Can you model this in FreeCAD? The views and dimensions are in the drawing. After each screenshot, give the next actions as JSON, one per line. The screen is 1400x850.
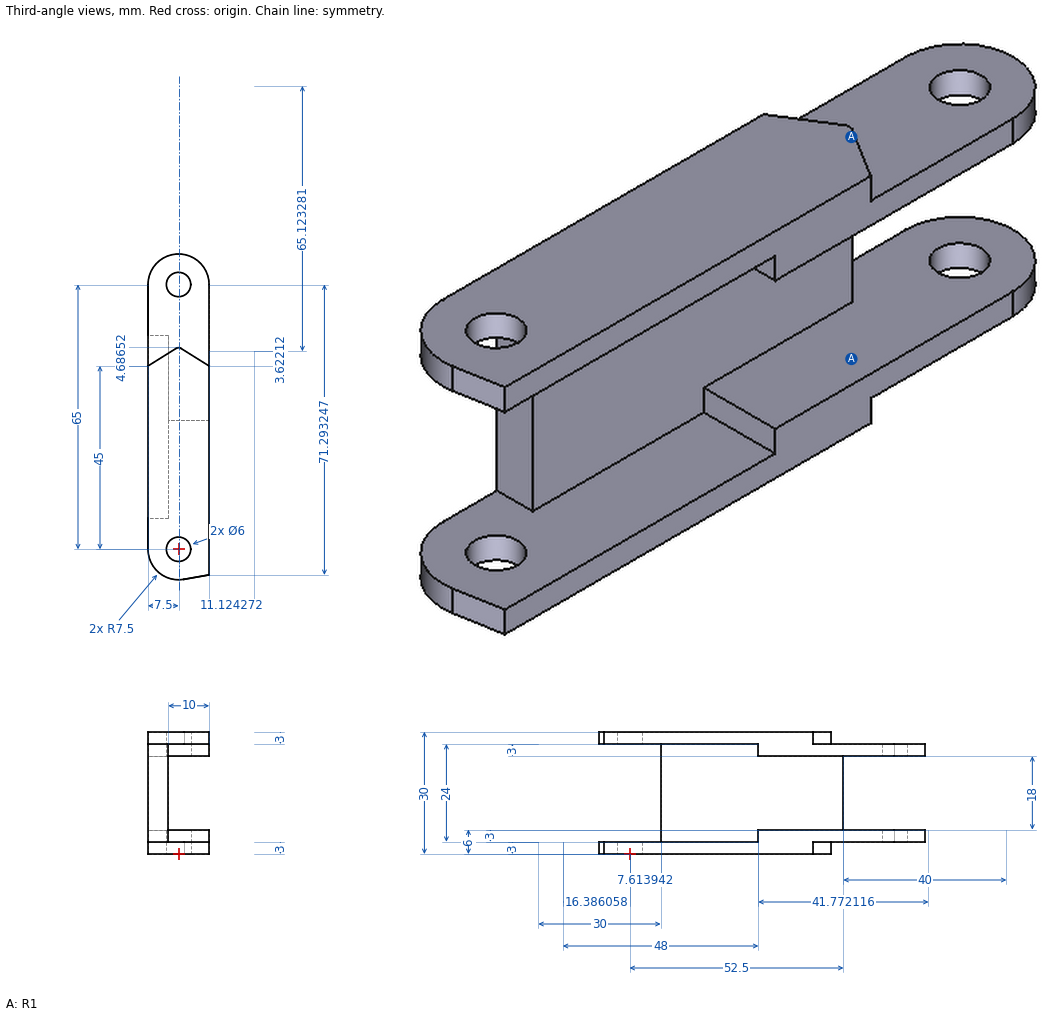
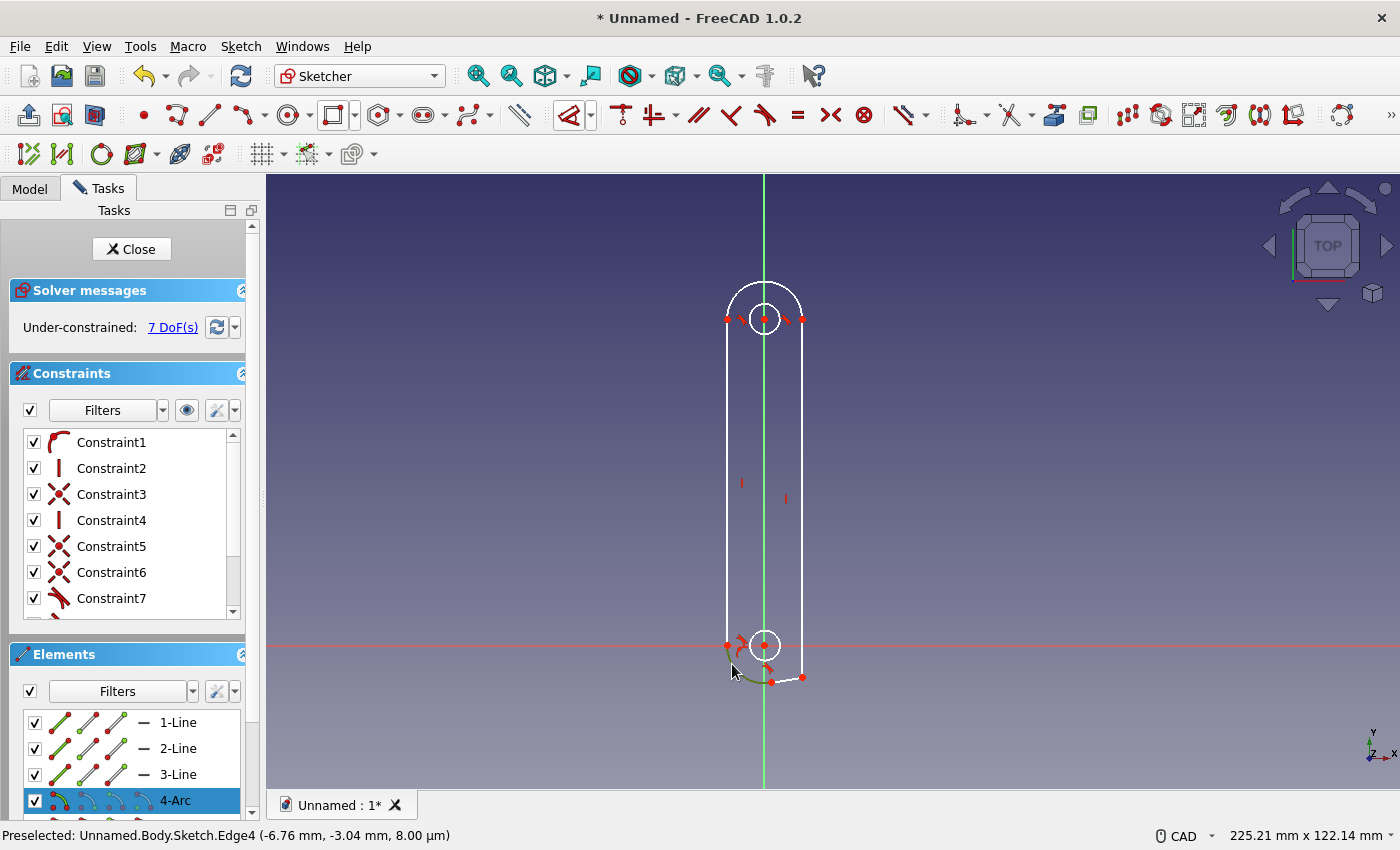
{"action": "left_click", "coordinate": [787, 289]}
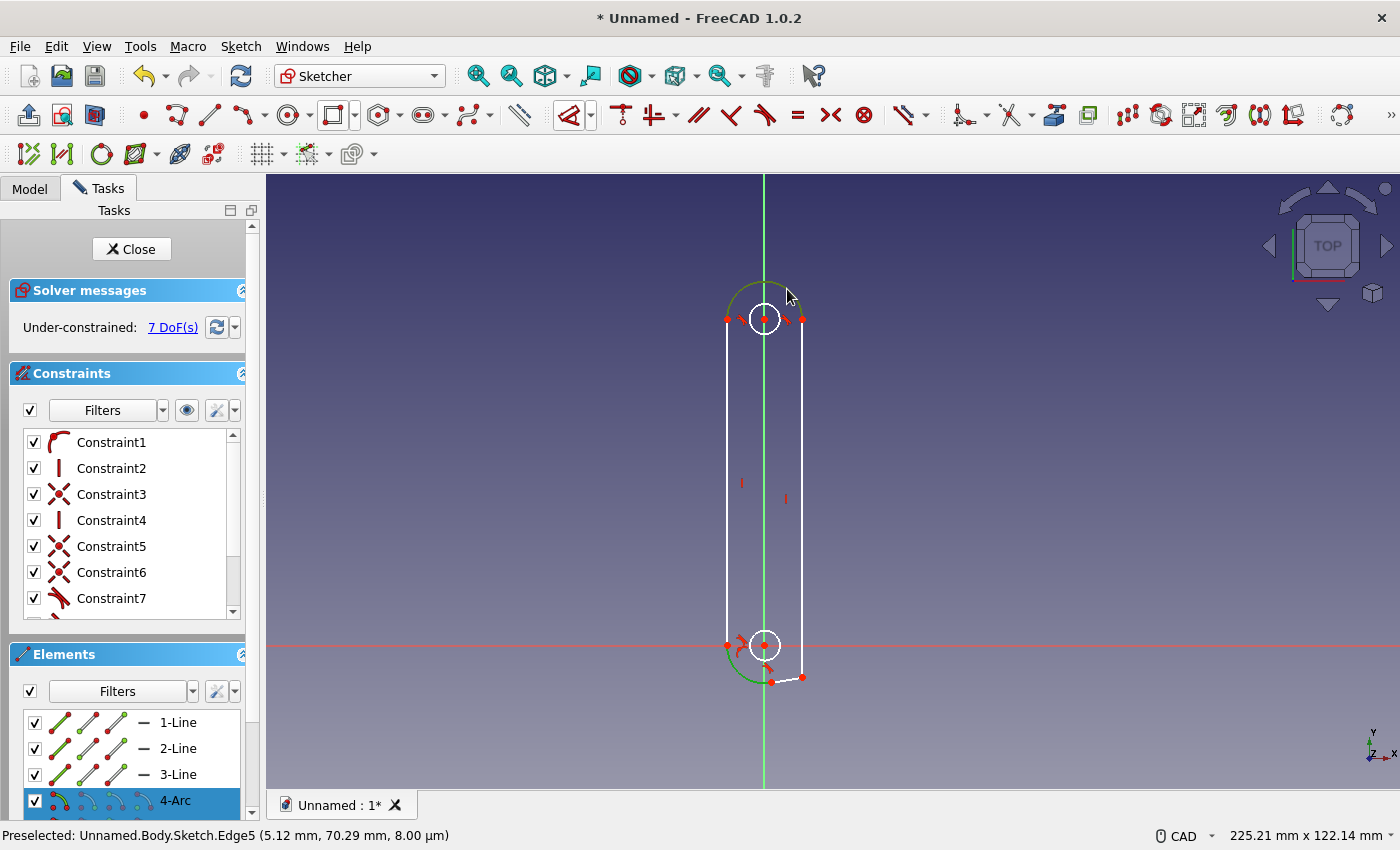
{"action": "key", "text": "e"}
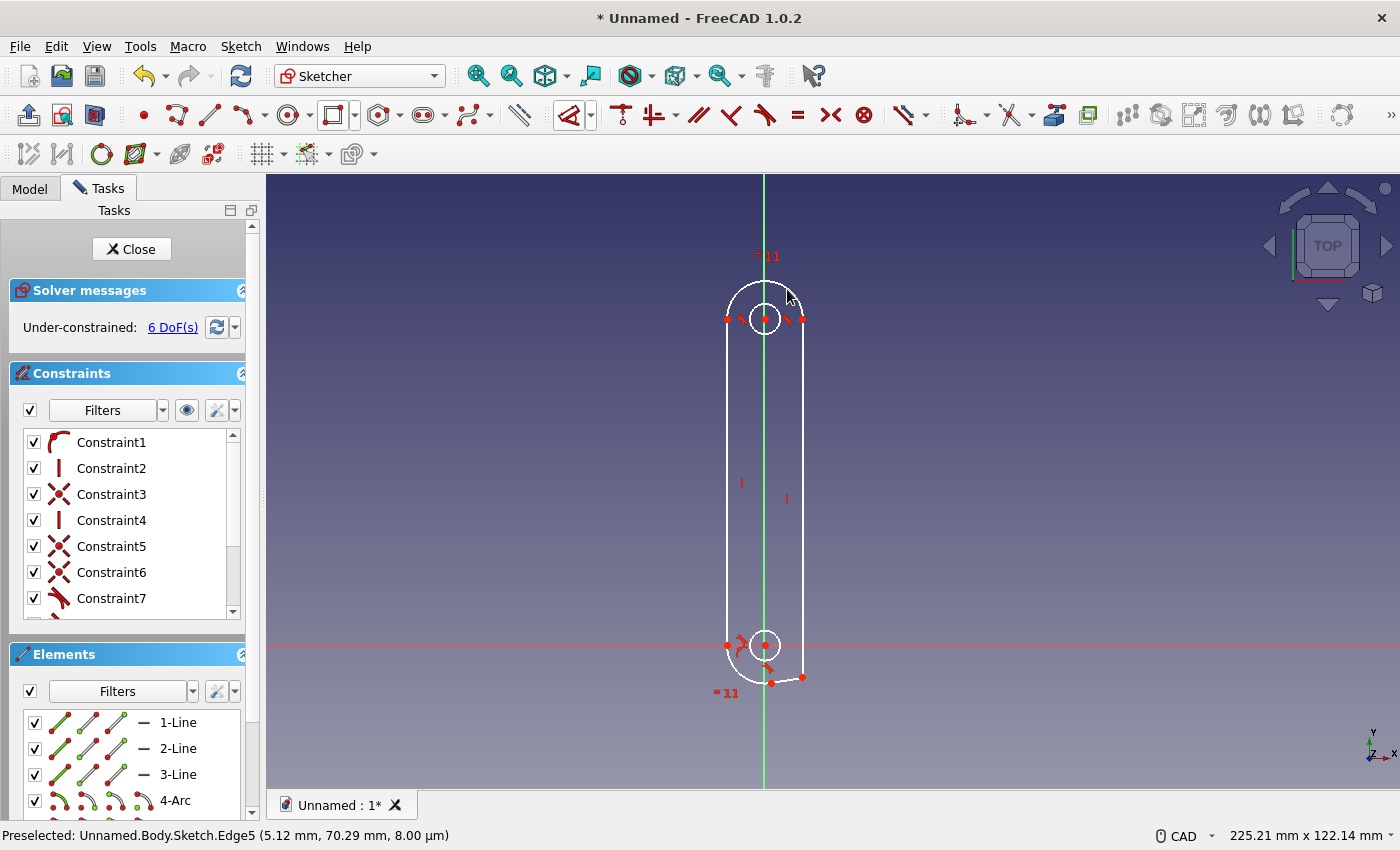
{"action": "scroll", "coordinate": [776, 635], "scroll_direction": "up", "scroll_amount": 2}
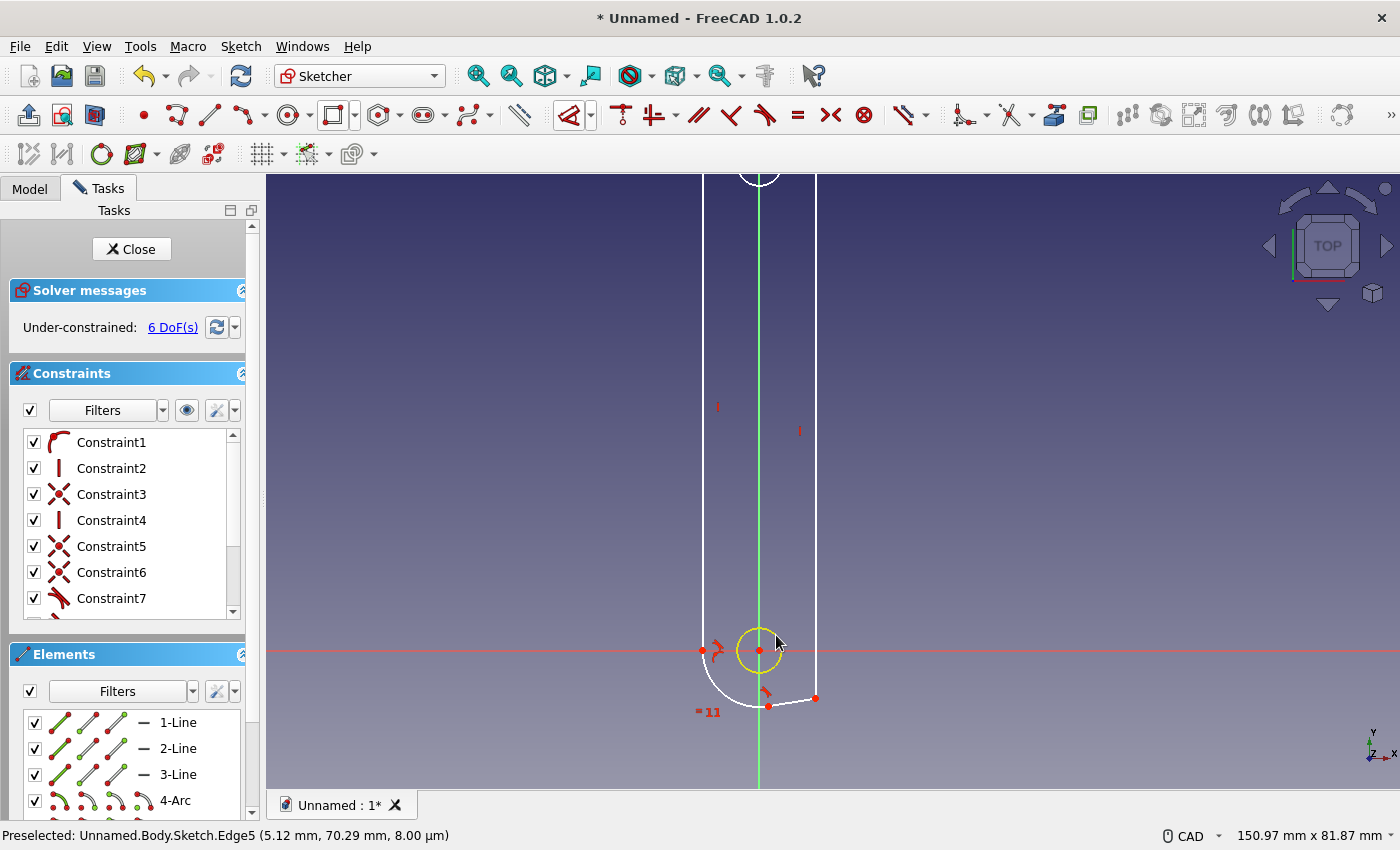
{"action": "left_click", "coordinate": [775, 635]}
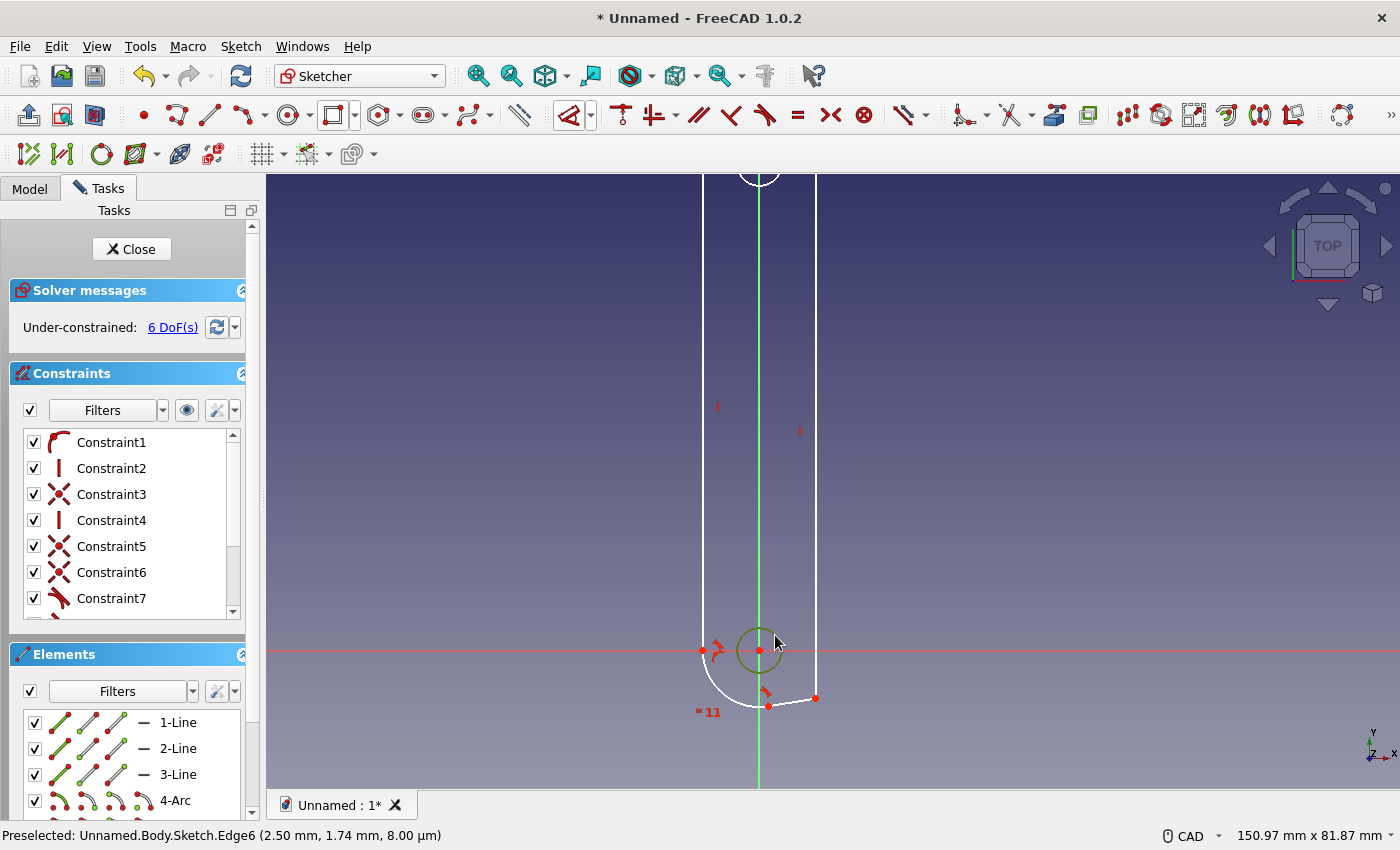
{"action": "scroll", "coordinate": [776, 635], "scroll_direction": "down", "scroll_amount": 2}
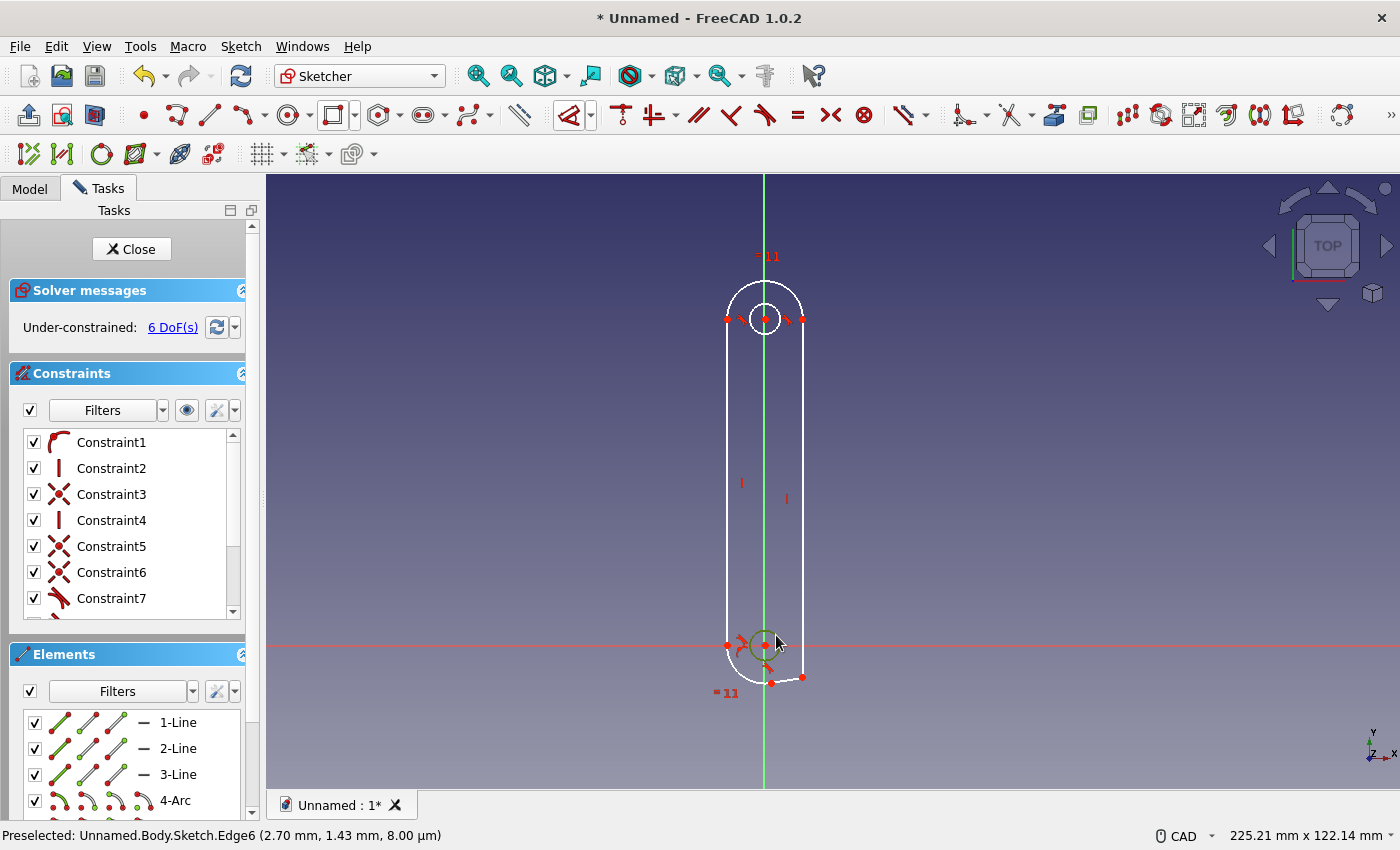
{"action": "scroll", "coordinate": [776, 308], "scroll_direction": "up", "scroll_amount": 2}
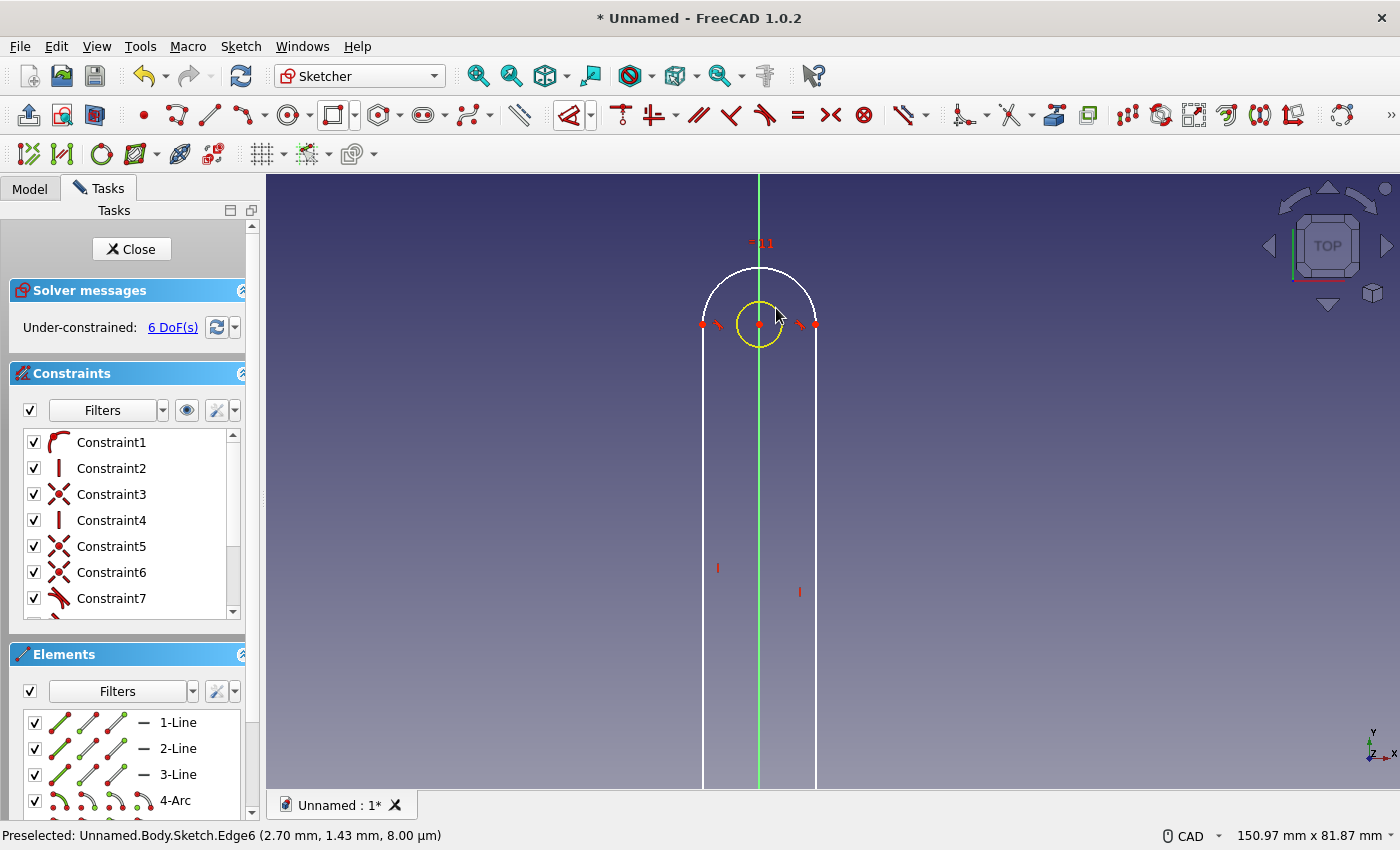
{"action": "left_click", "coordinate": [775, 308]}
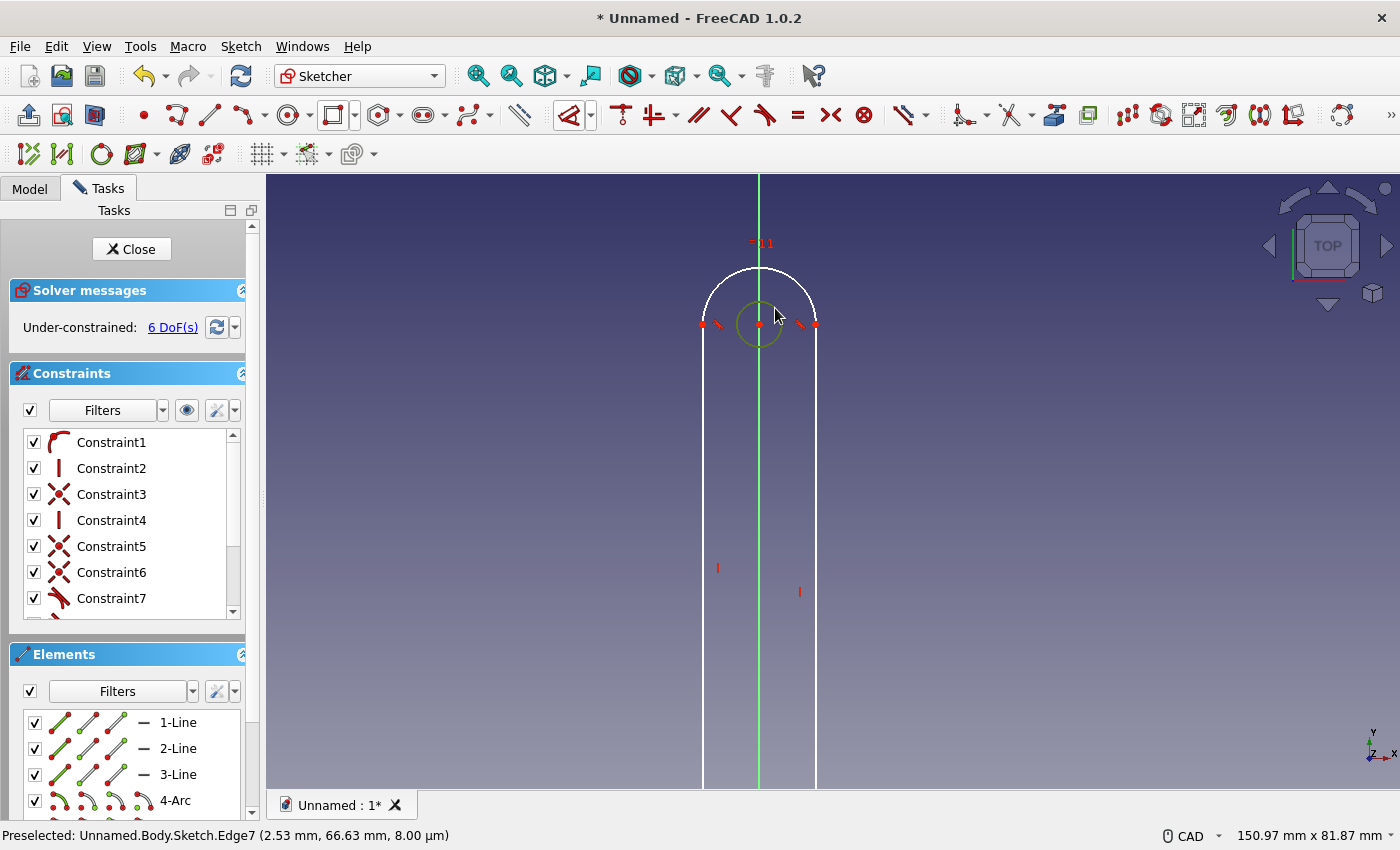
{"action": "key", "text": "e"}